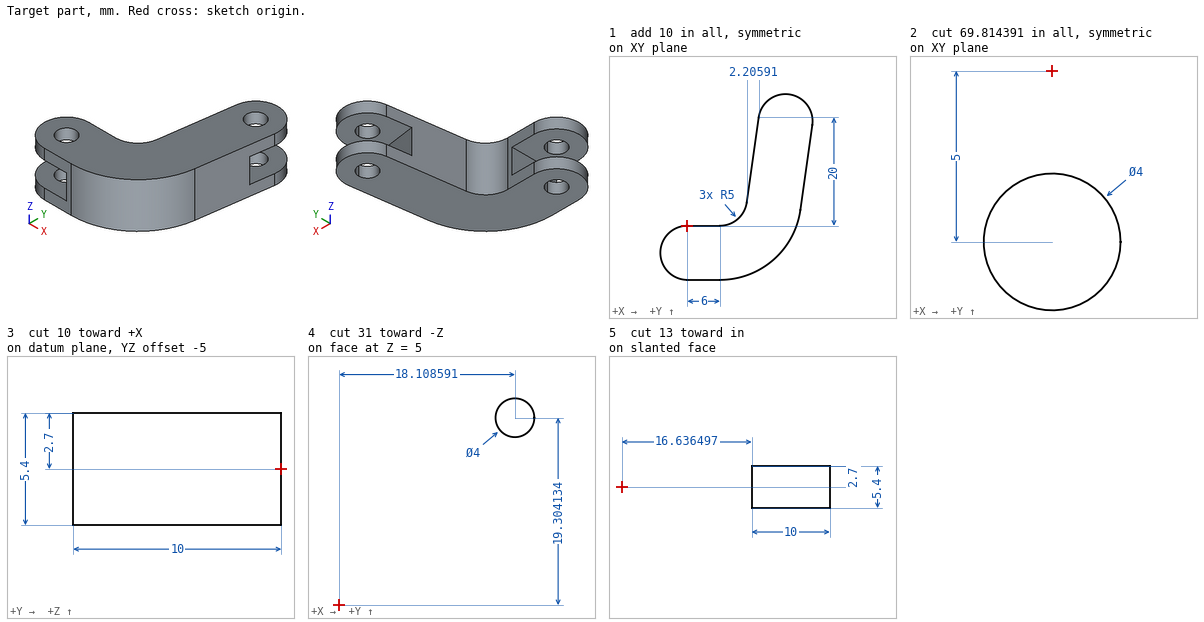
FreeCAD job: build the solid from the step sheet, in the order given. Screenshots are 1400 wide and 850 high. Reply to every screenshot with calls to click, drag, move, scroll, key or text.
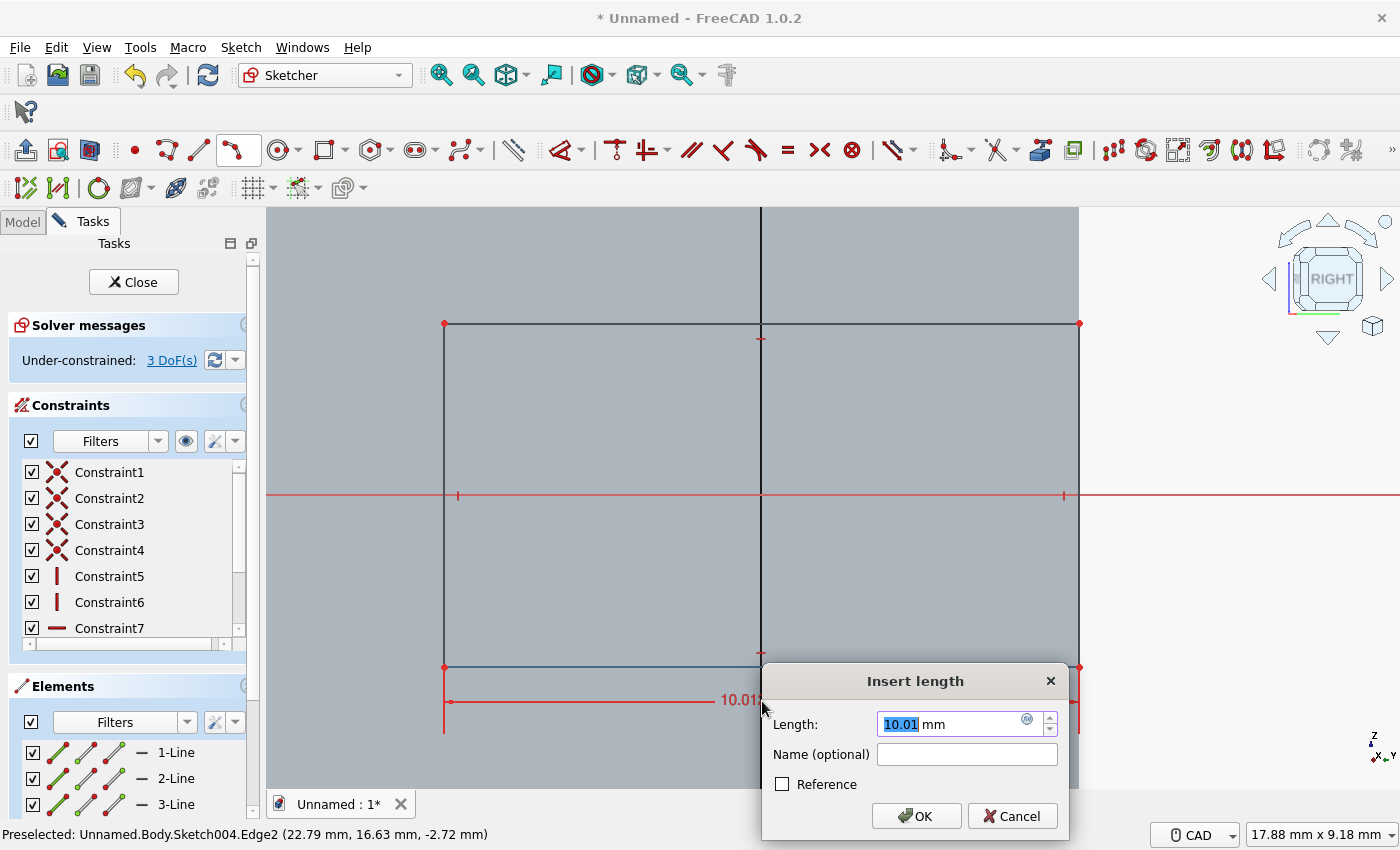
text(10)
key(Return)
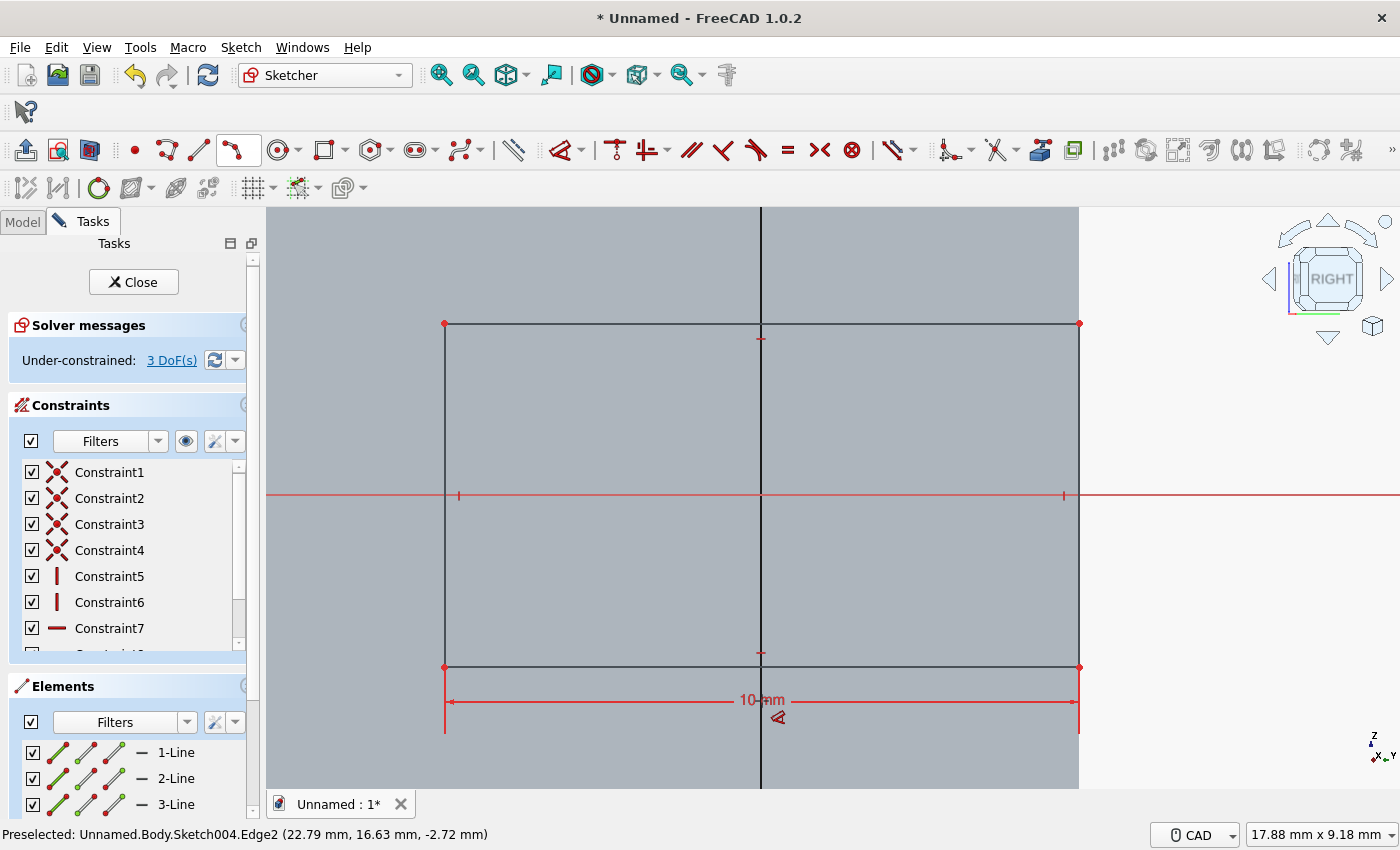
click(445, 427)
click(411, 417)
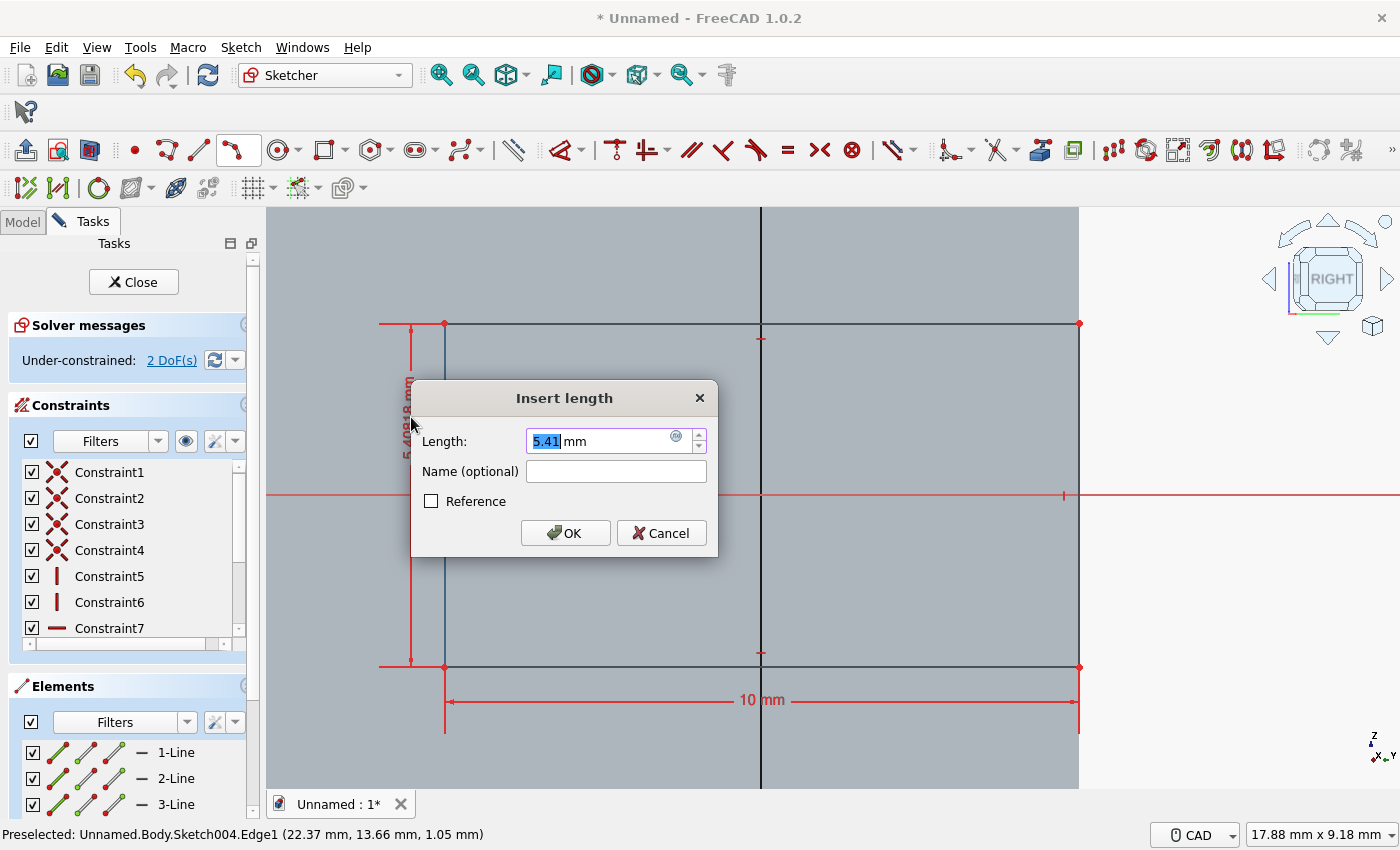
text(5.4)
key(Return)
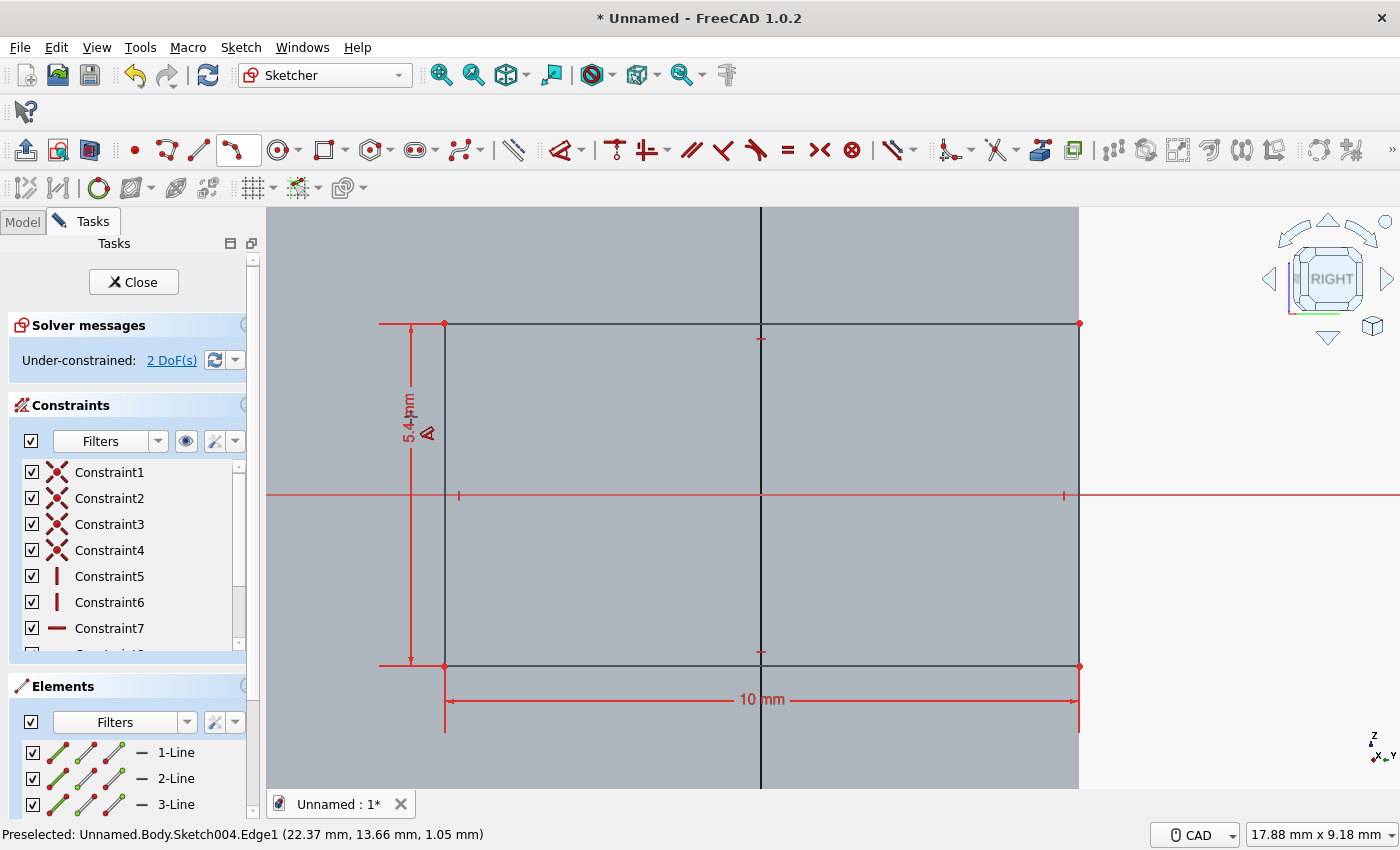
click(445, 324)
click(479, 370)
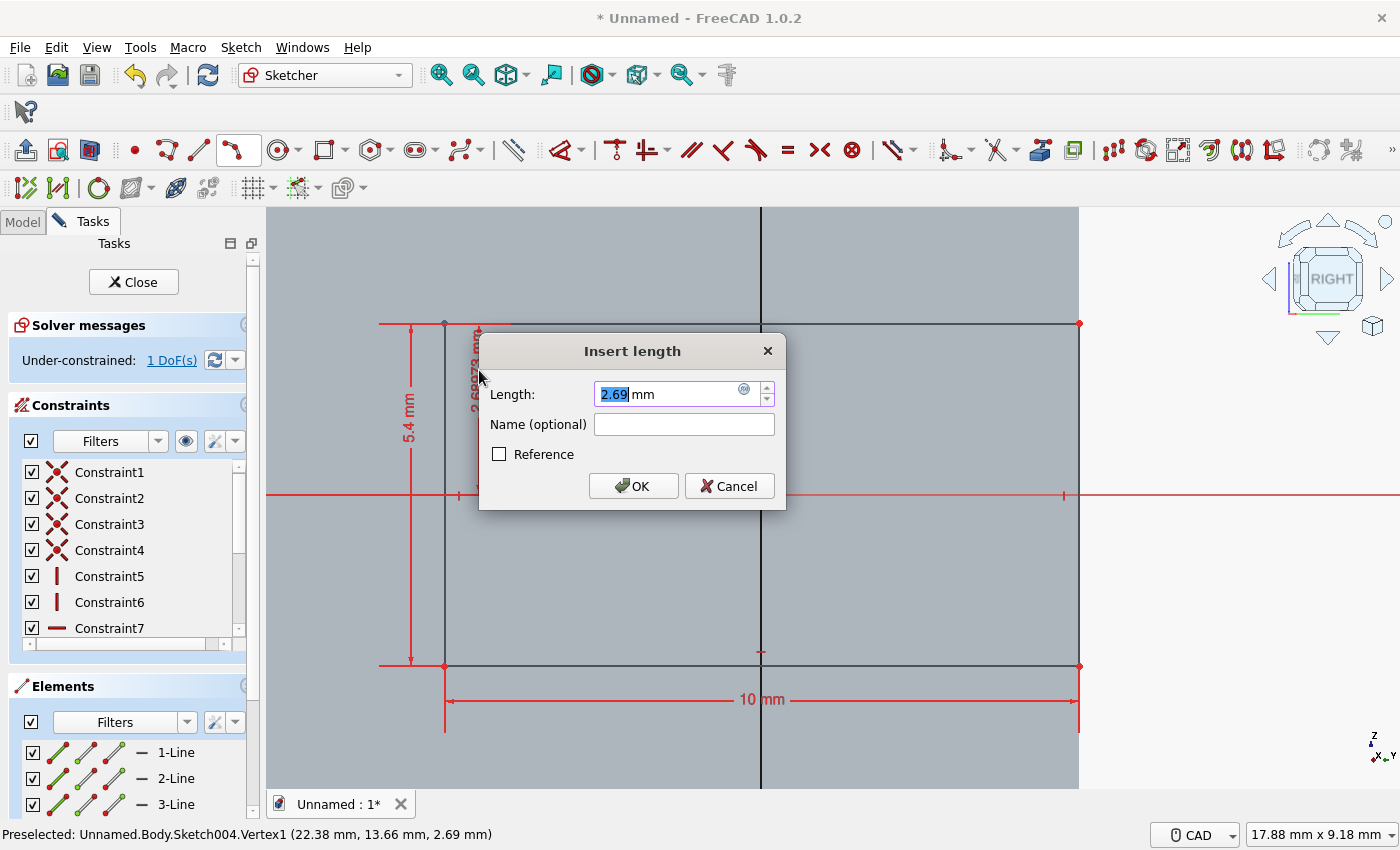
text(2.7)
key(Return)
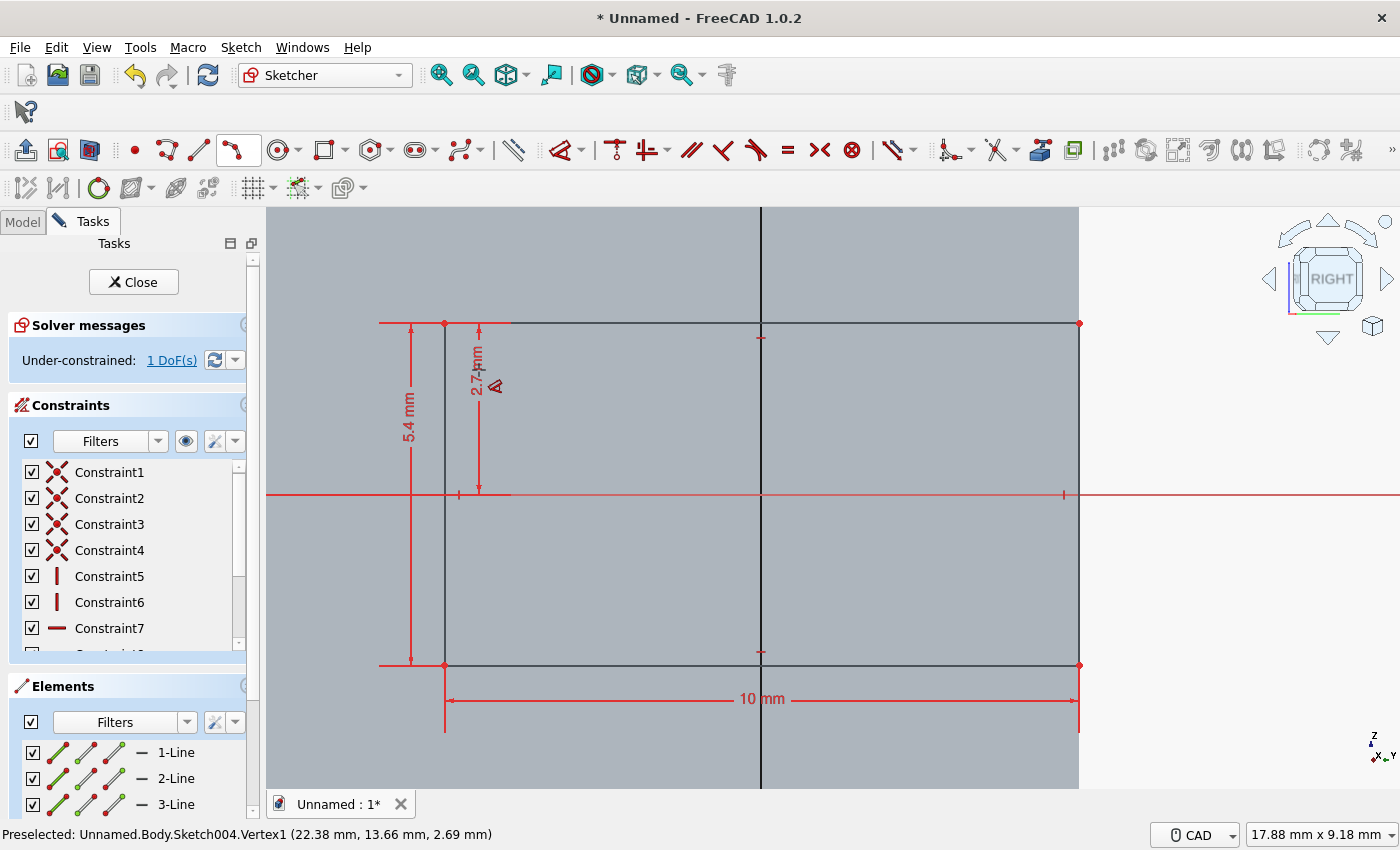
click(445, 323)
click(369, 289)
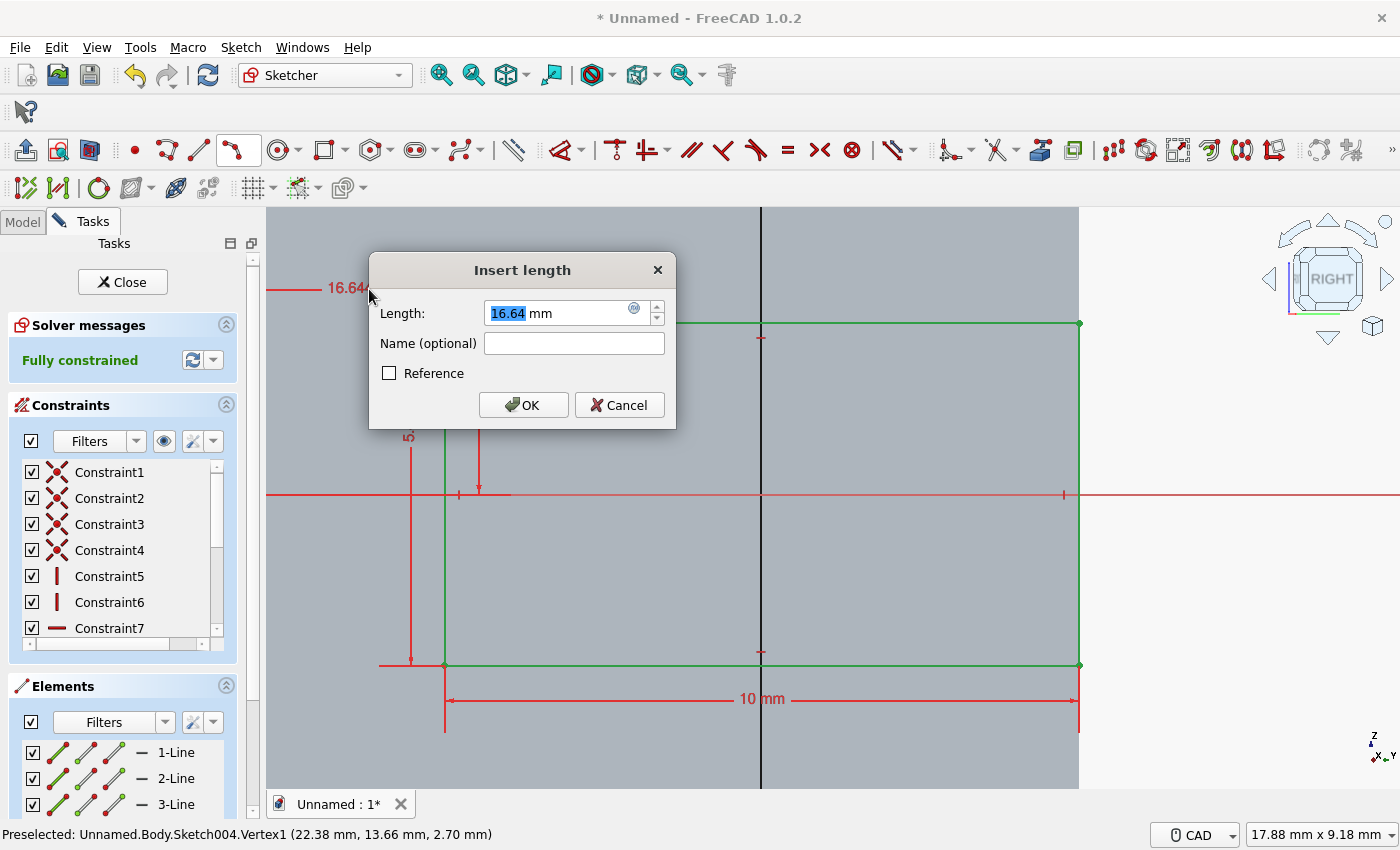
text(16.636497)
key(Return)
key(Escape)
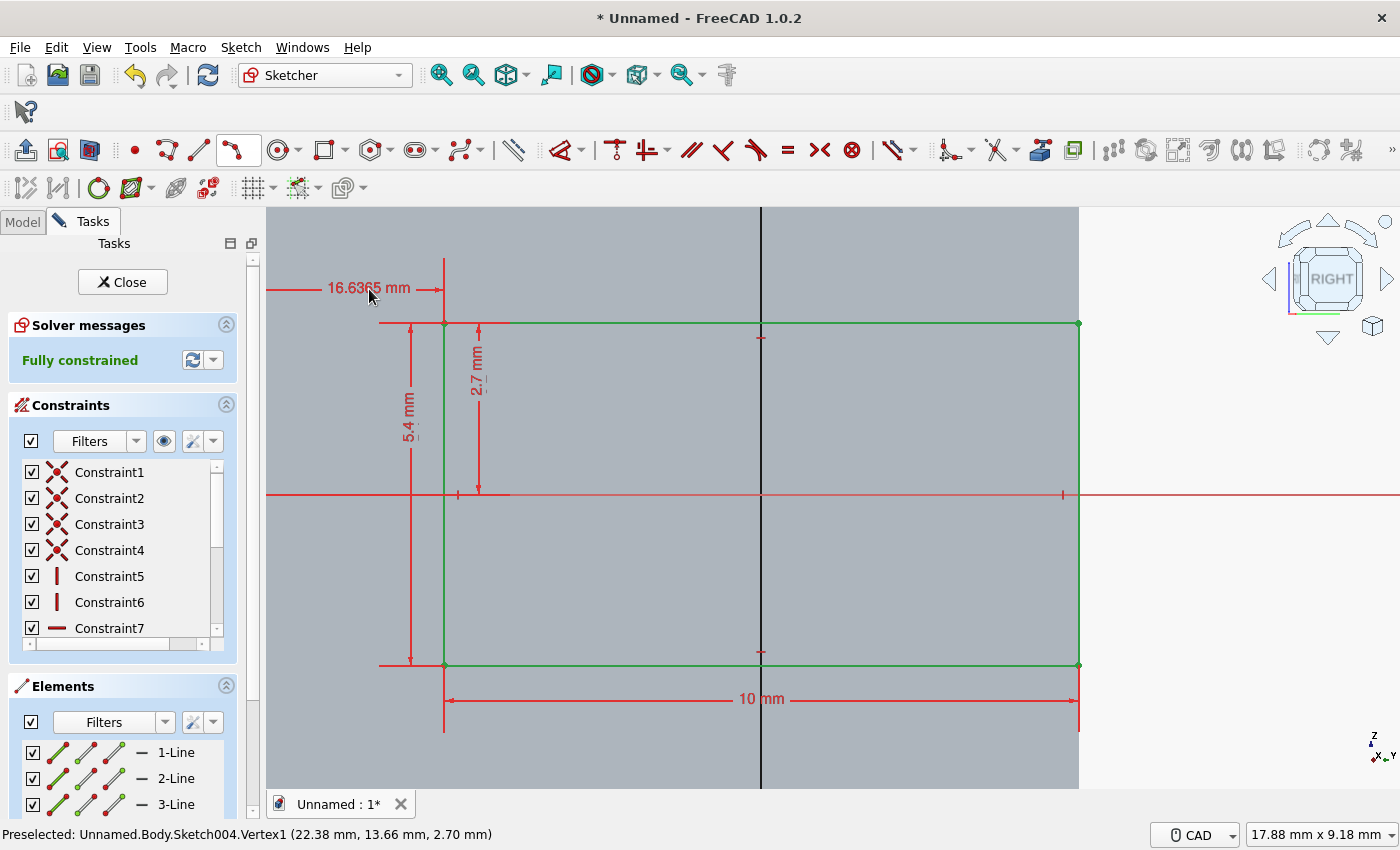
click(123, 282)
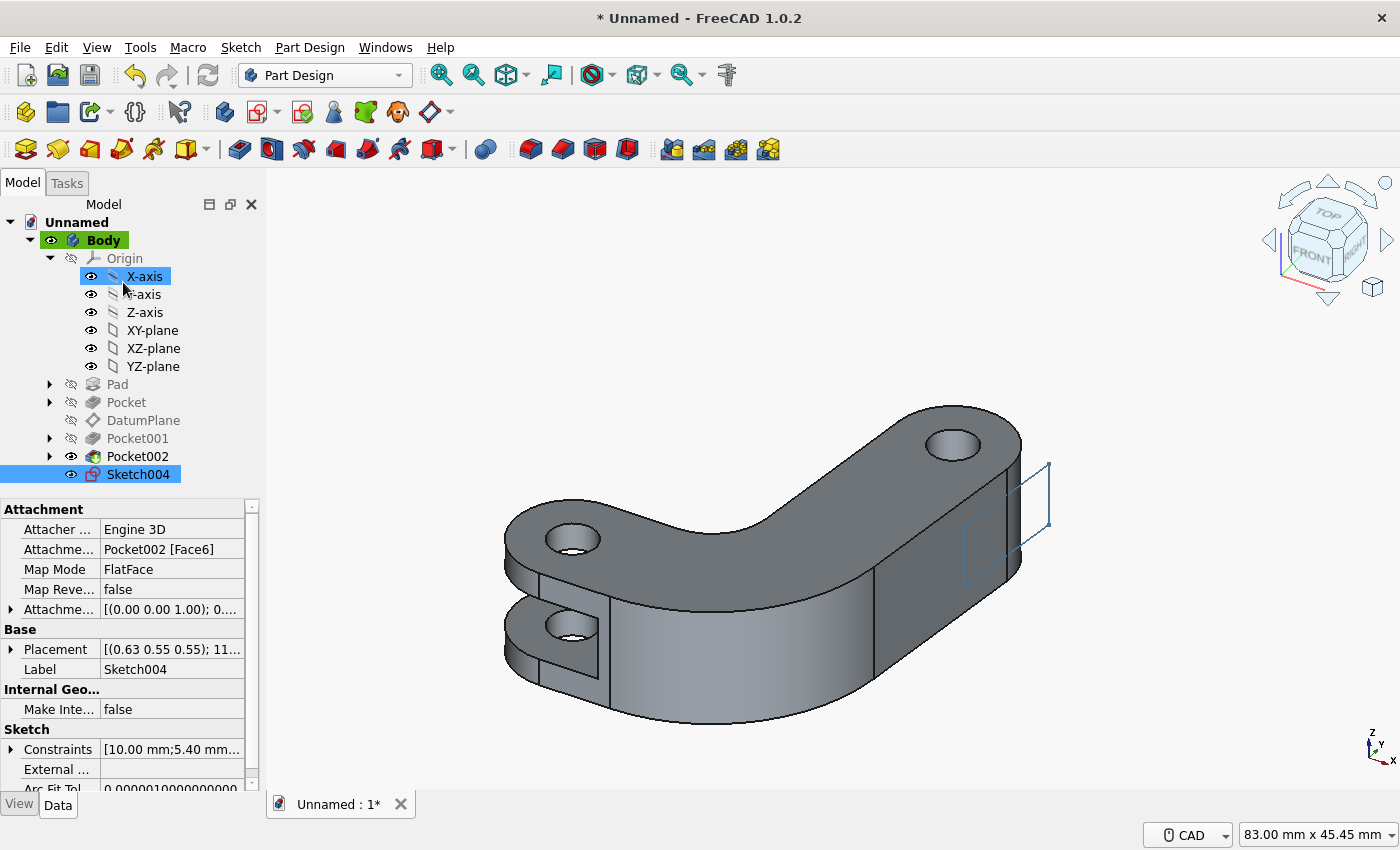
click(240, 150)